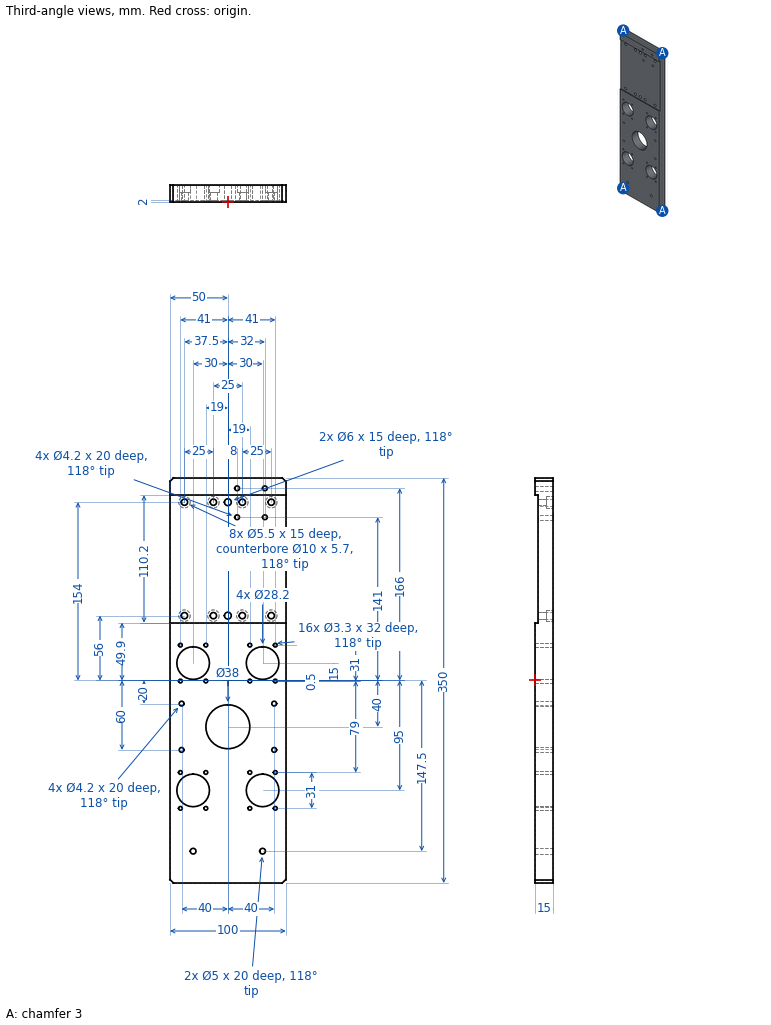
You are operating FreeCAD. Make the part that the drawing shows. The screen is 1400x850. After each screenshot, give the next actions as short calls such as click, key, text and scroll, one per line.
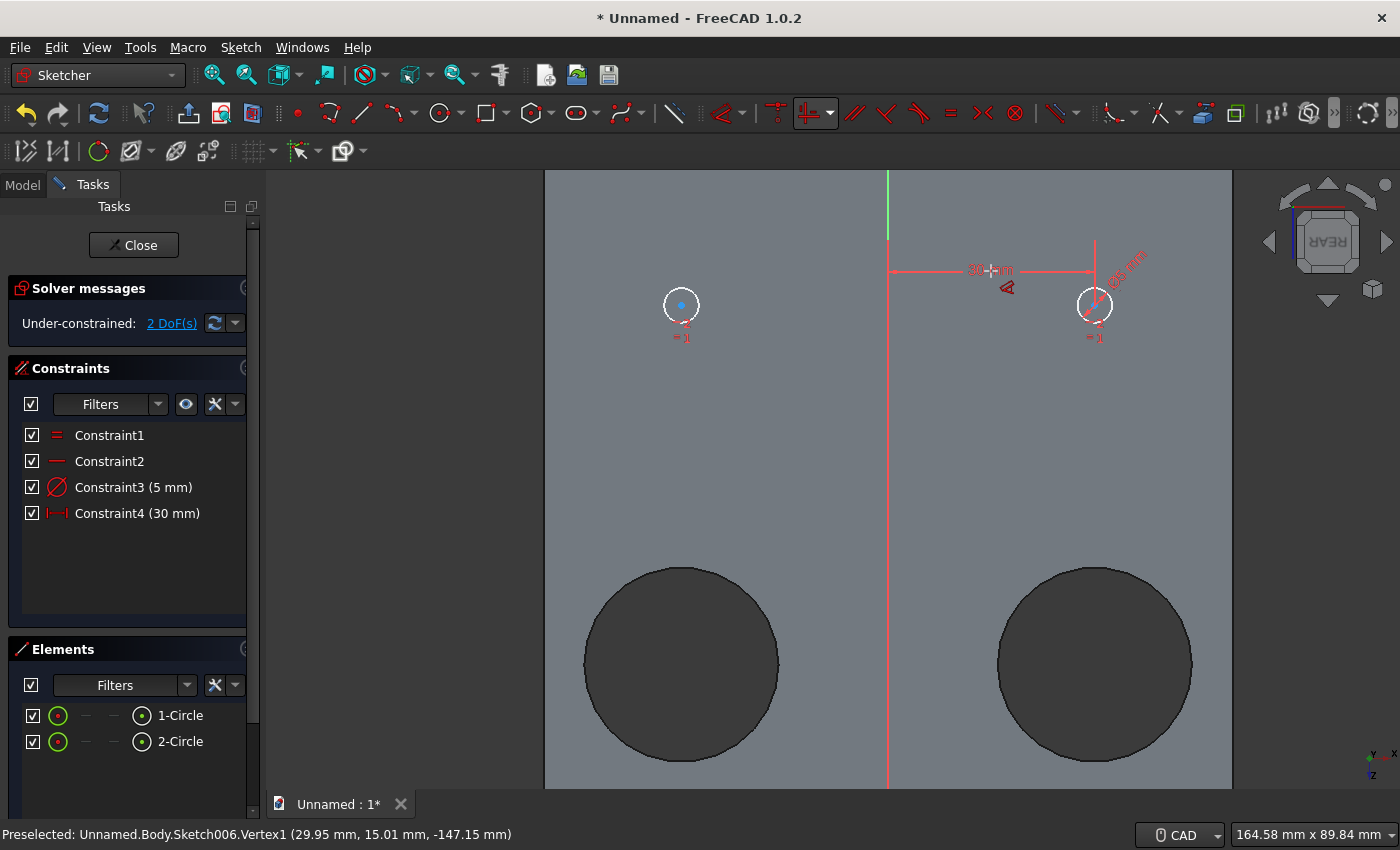
click(681, 305)
click(785, 271)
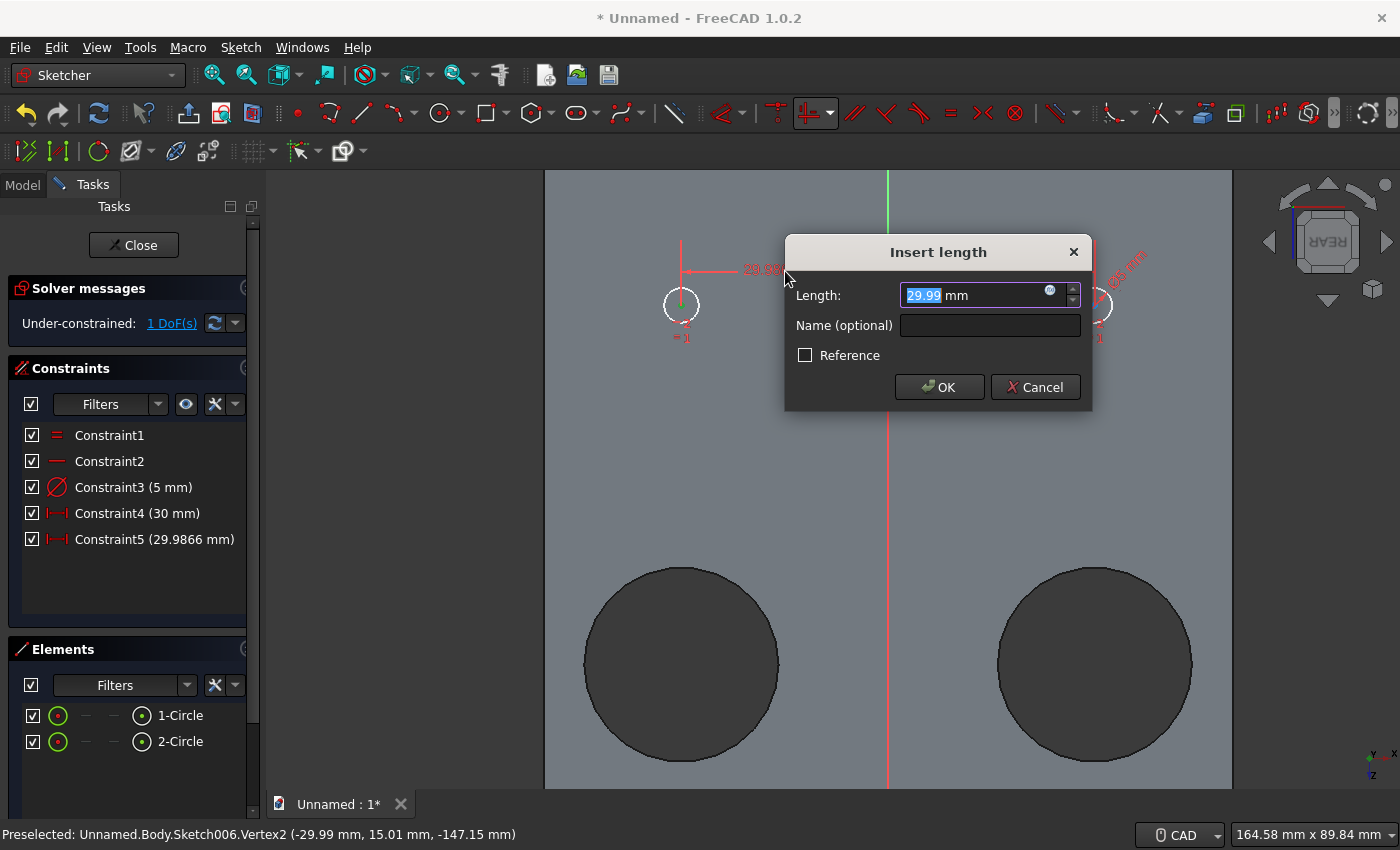
text(30)
key(Return)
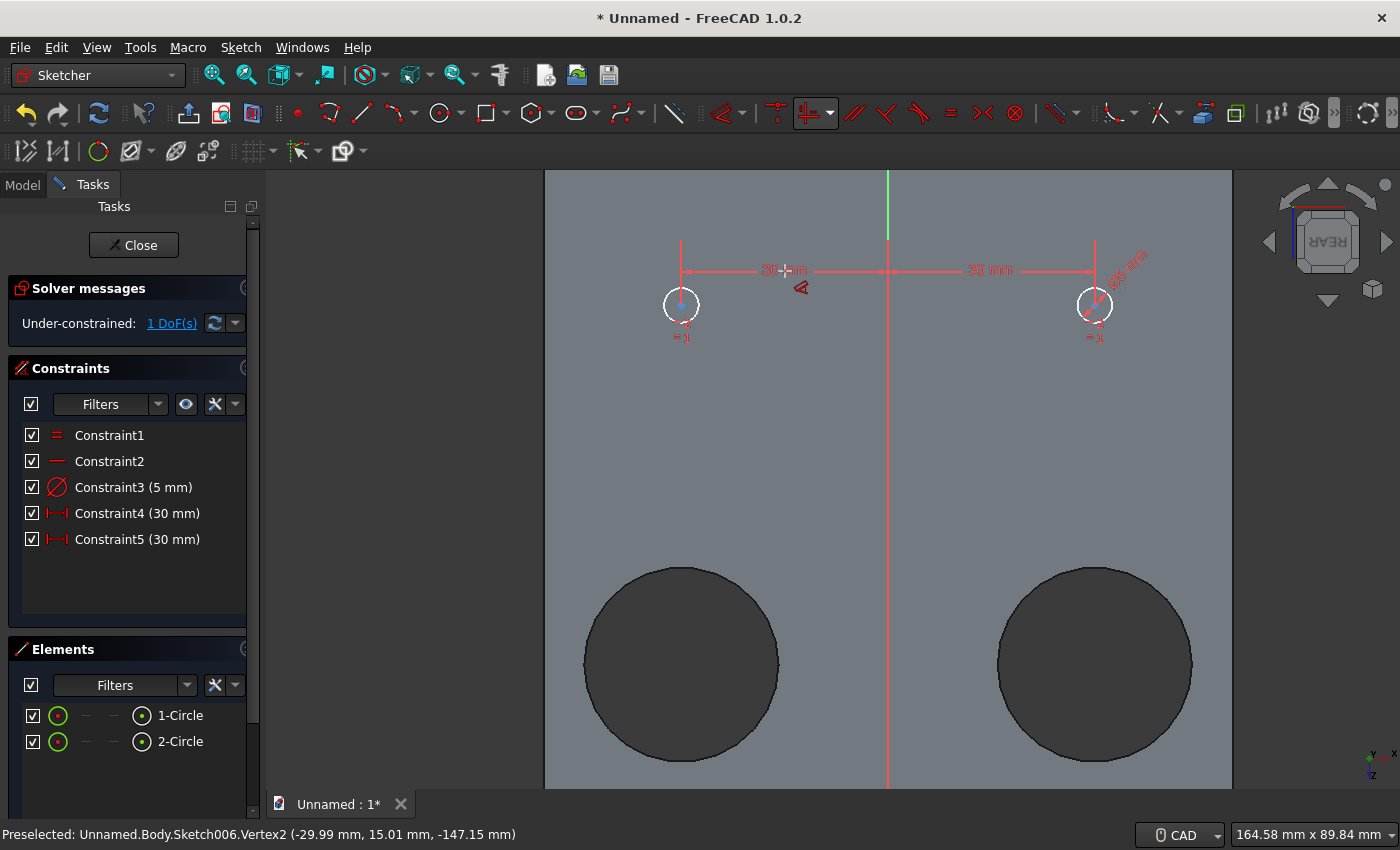
click(1095, 305)
click(1129, 533)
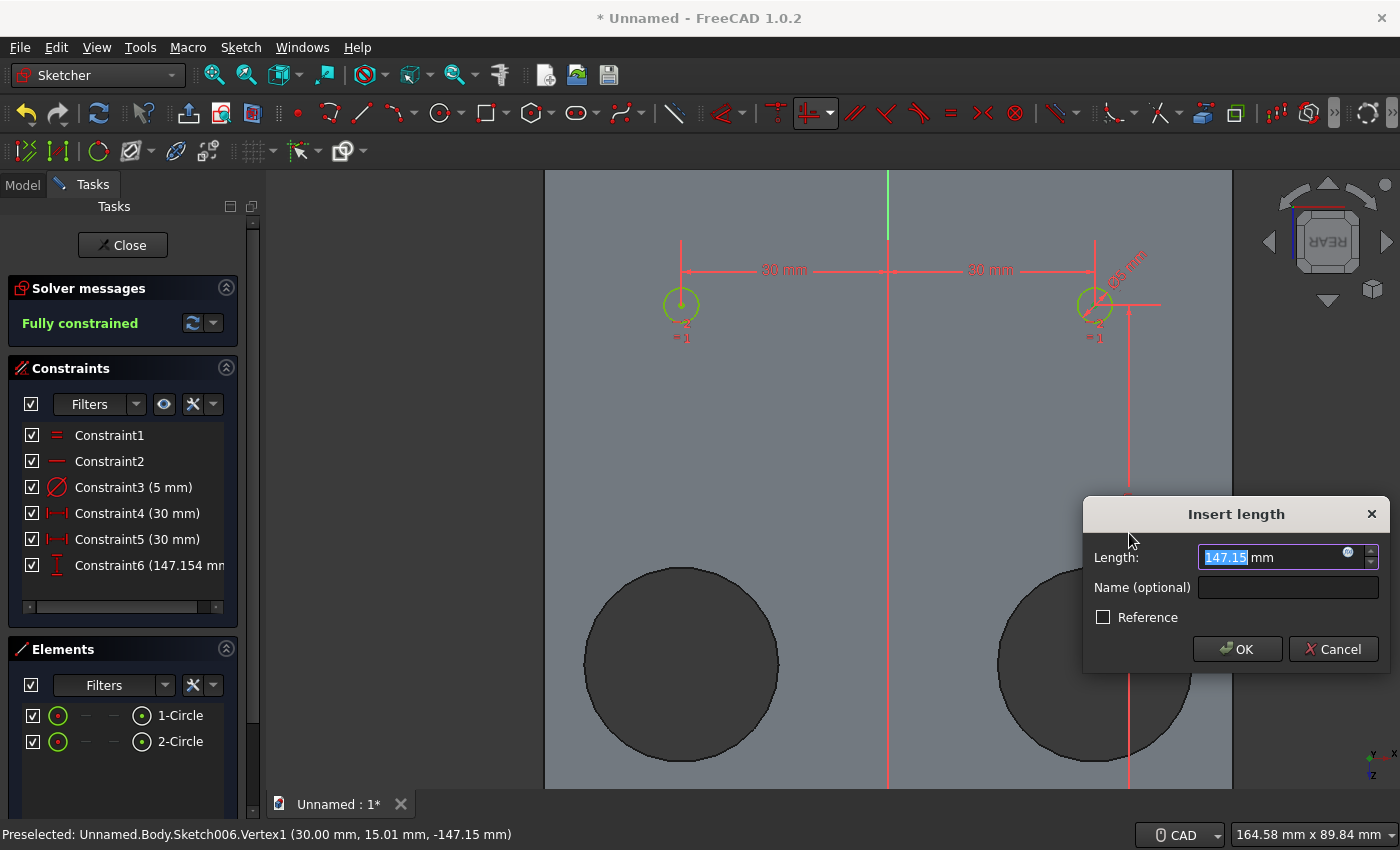
text(147.5)
key(Return)
key(Escape)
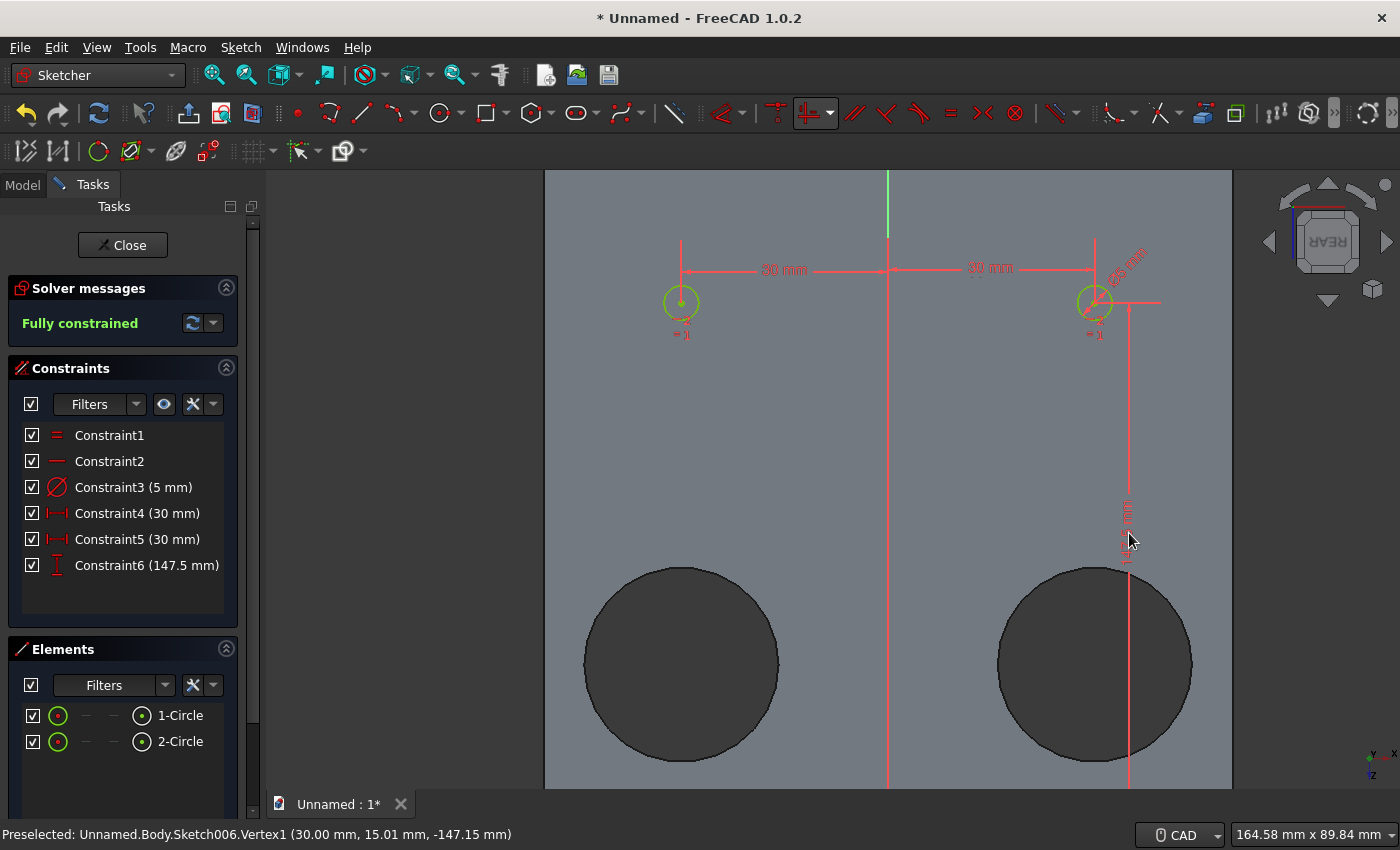
click(123, 245)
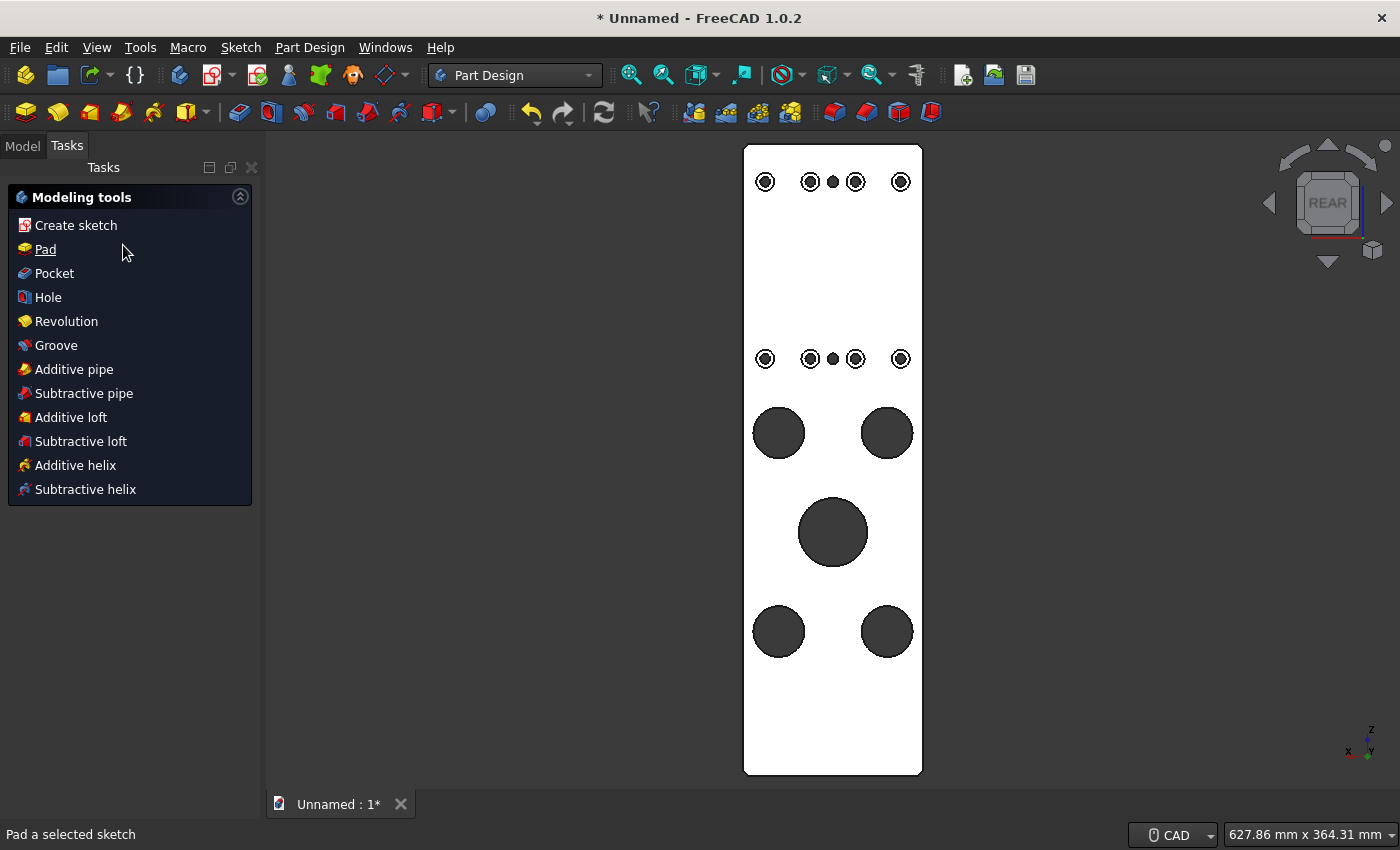
click(272, 112)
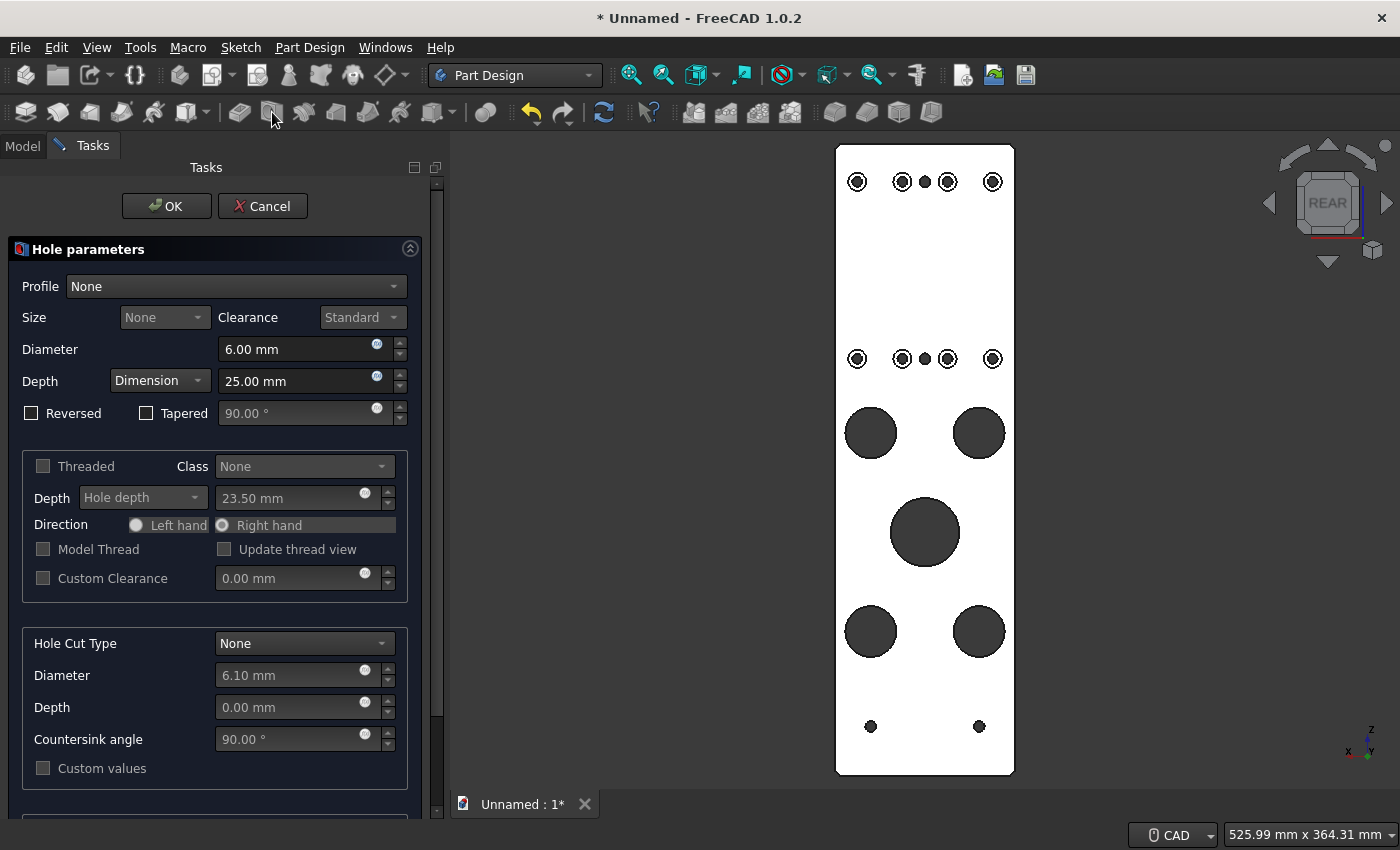
triple_click(305, 349)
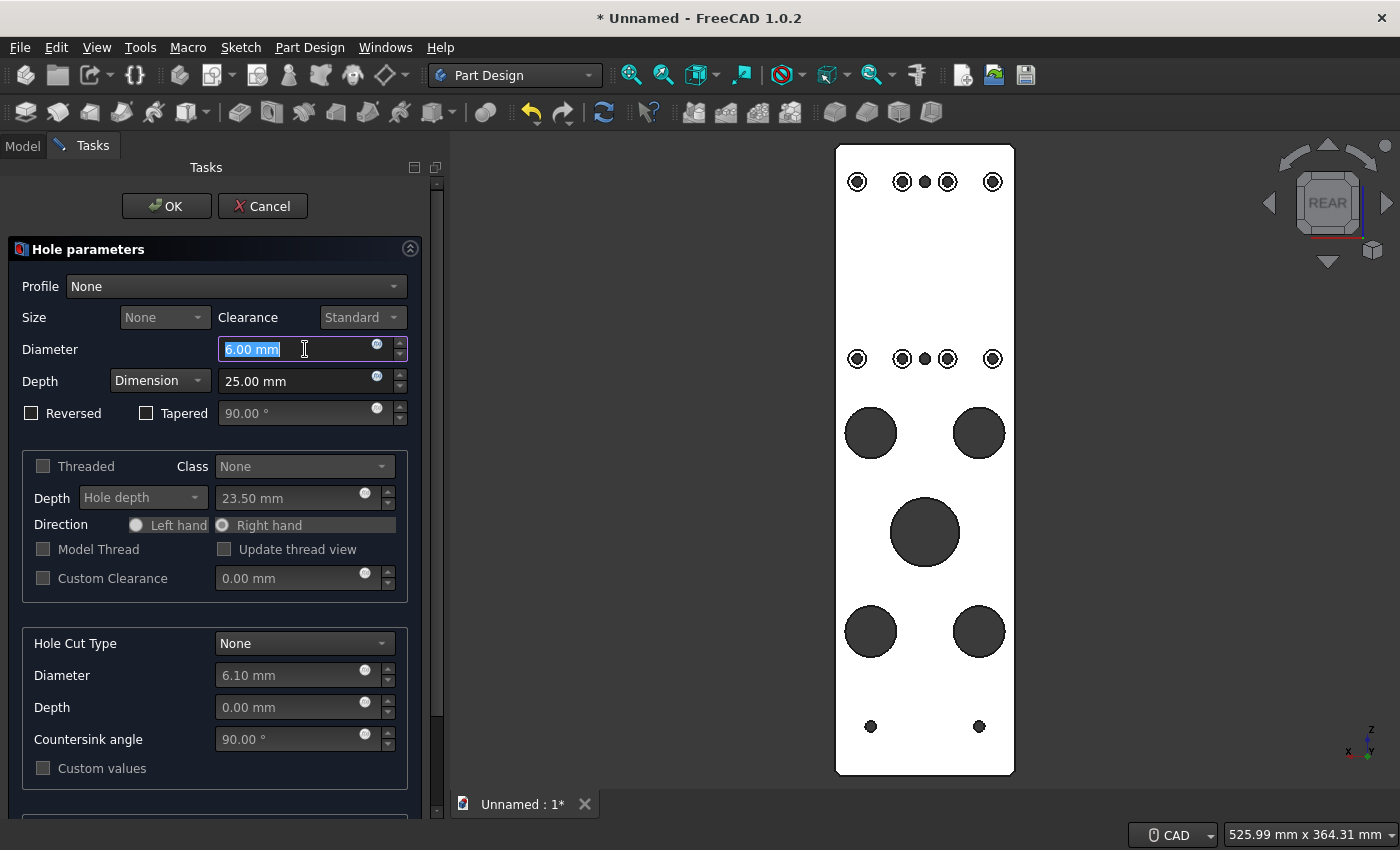
text(5)
key(Tab)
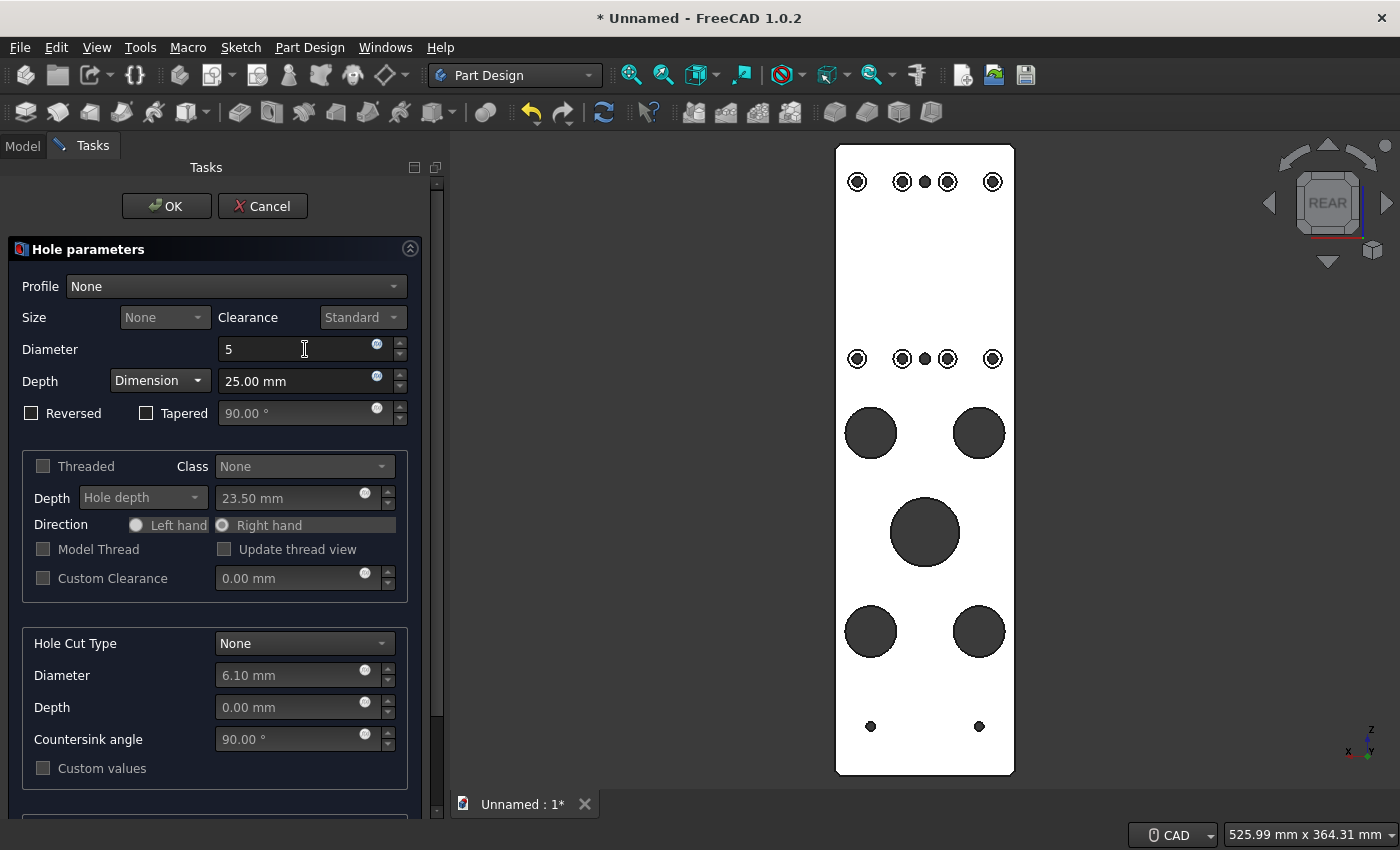
triple_click(305, 381)